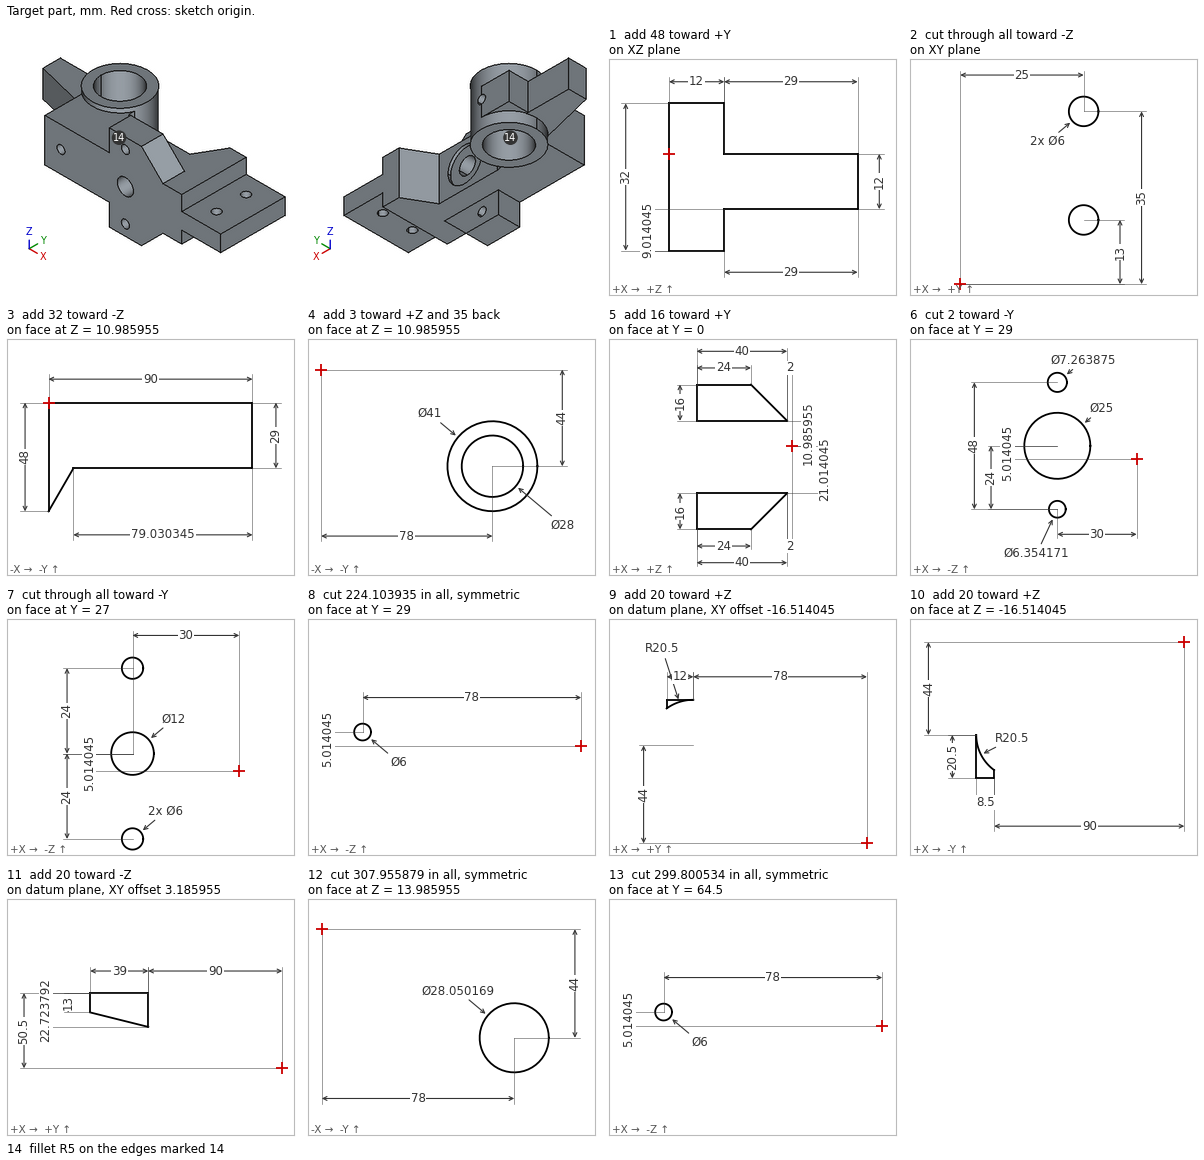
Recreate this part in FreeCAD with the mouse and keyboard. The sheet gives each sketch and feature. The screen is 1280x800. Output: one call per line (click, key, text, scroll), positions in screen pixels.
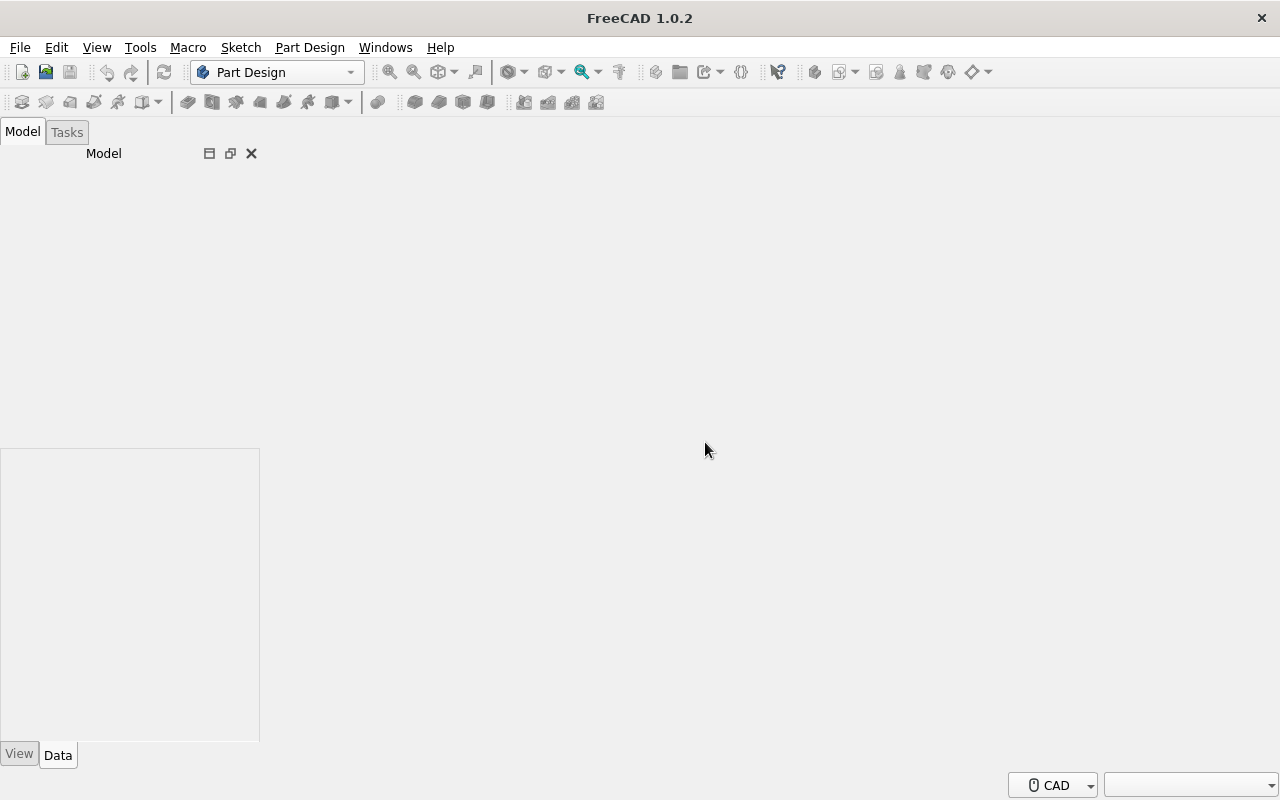
click(22, 72)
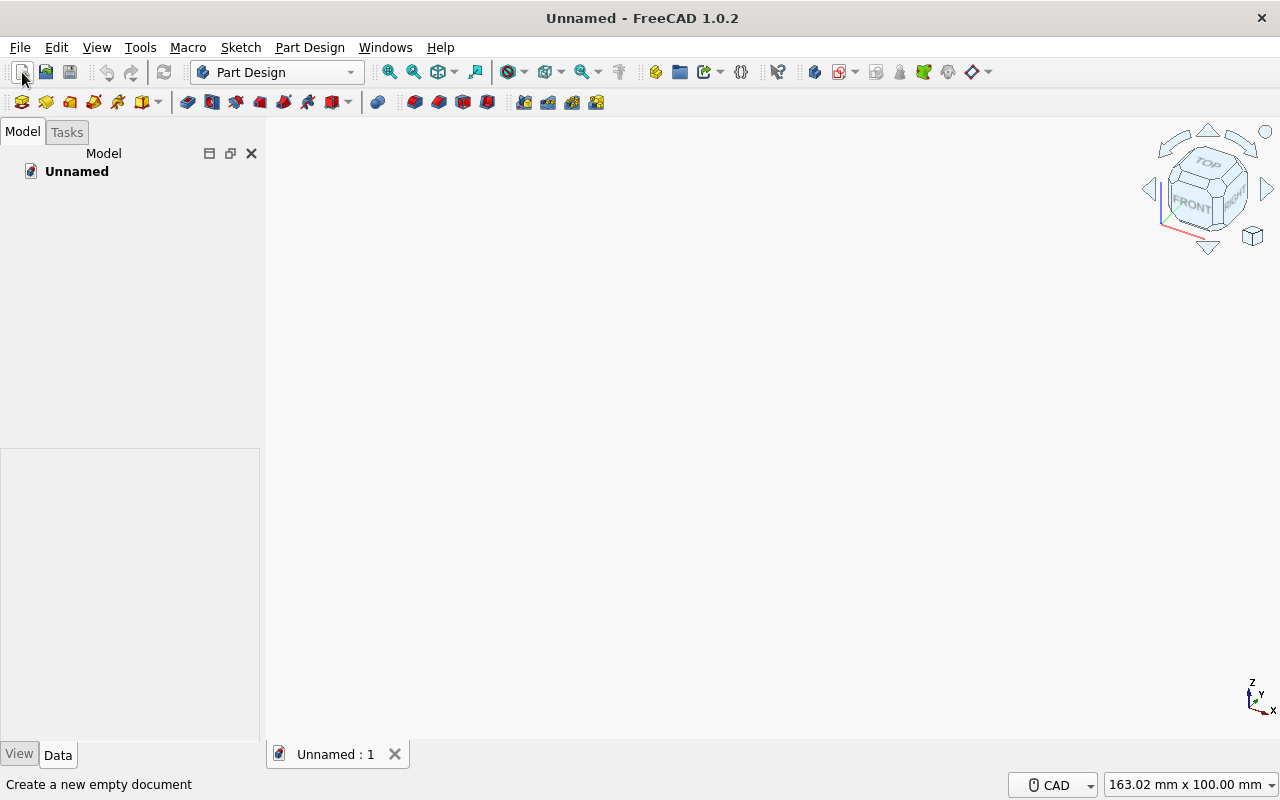
click(840, 72)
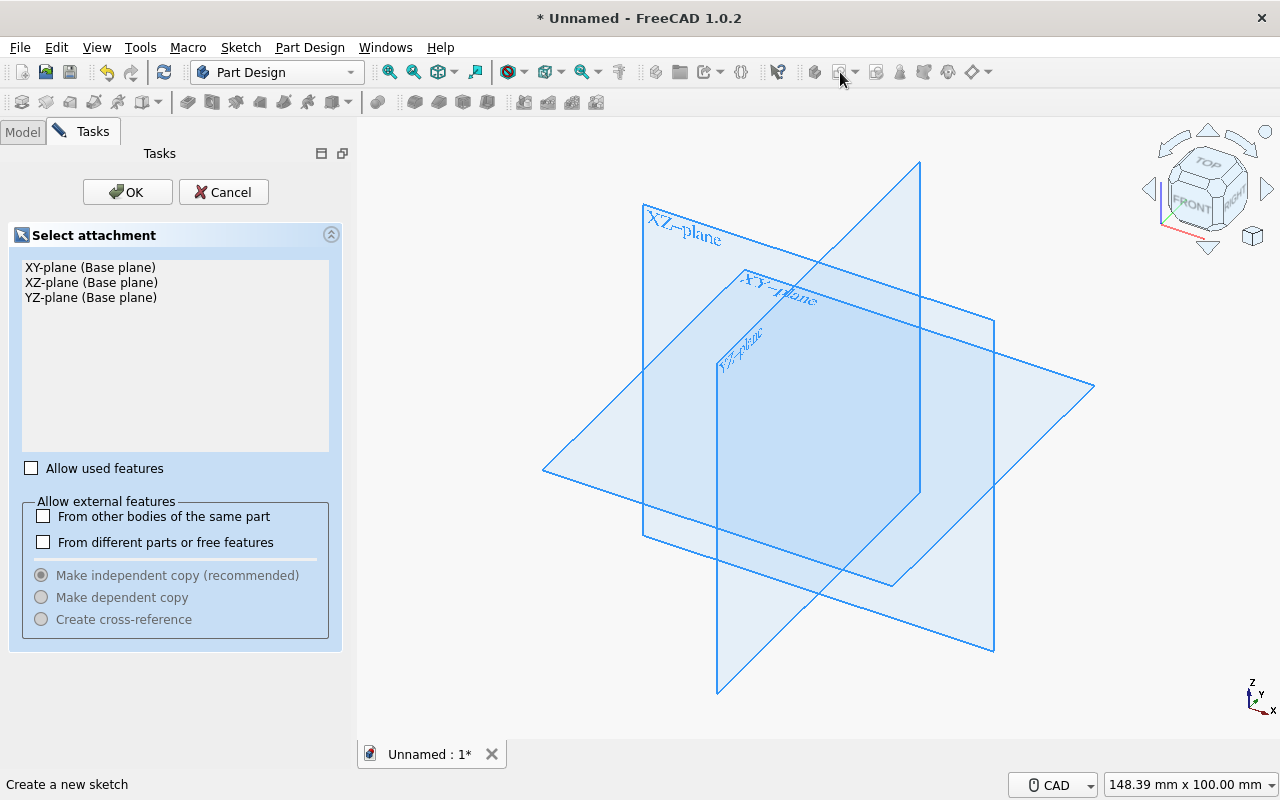
click(82, 282)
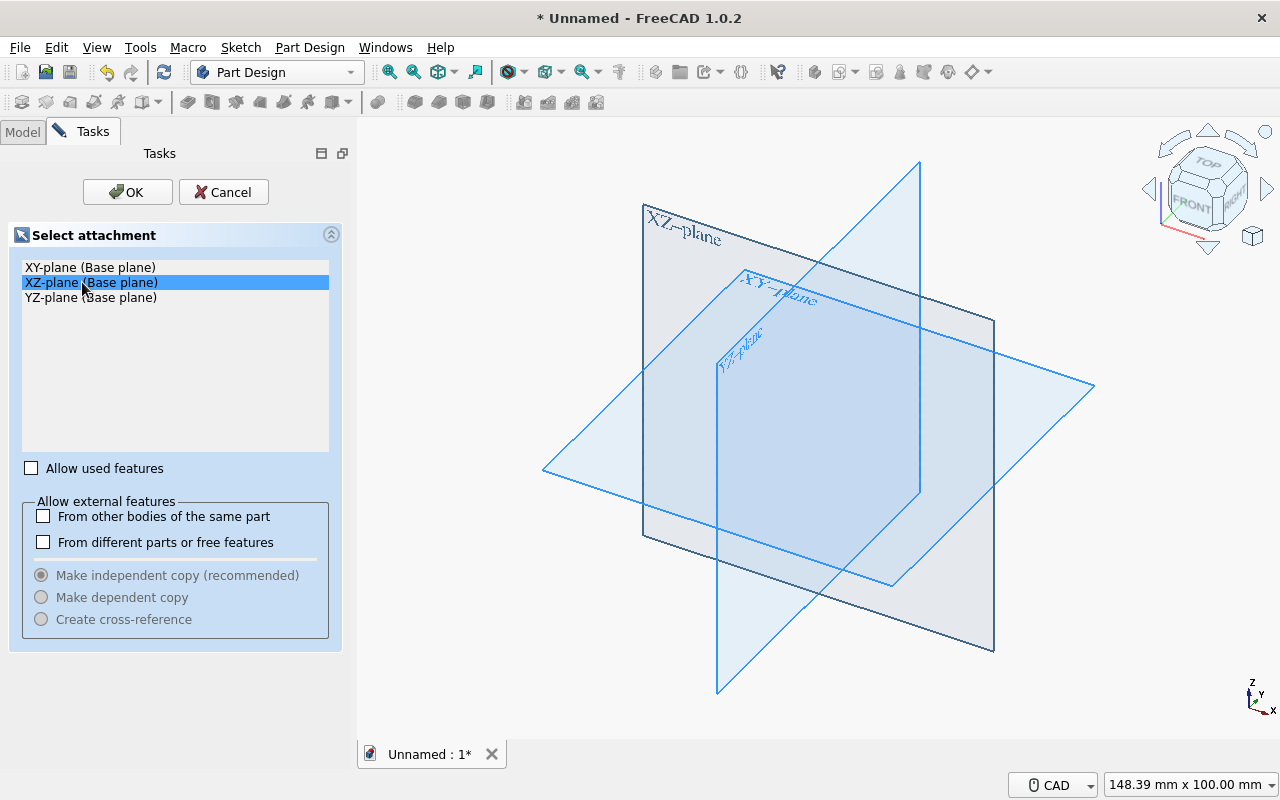
click(128, 192)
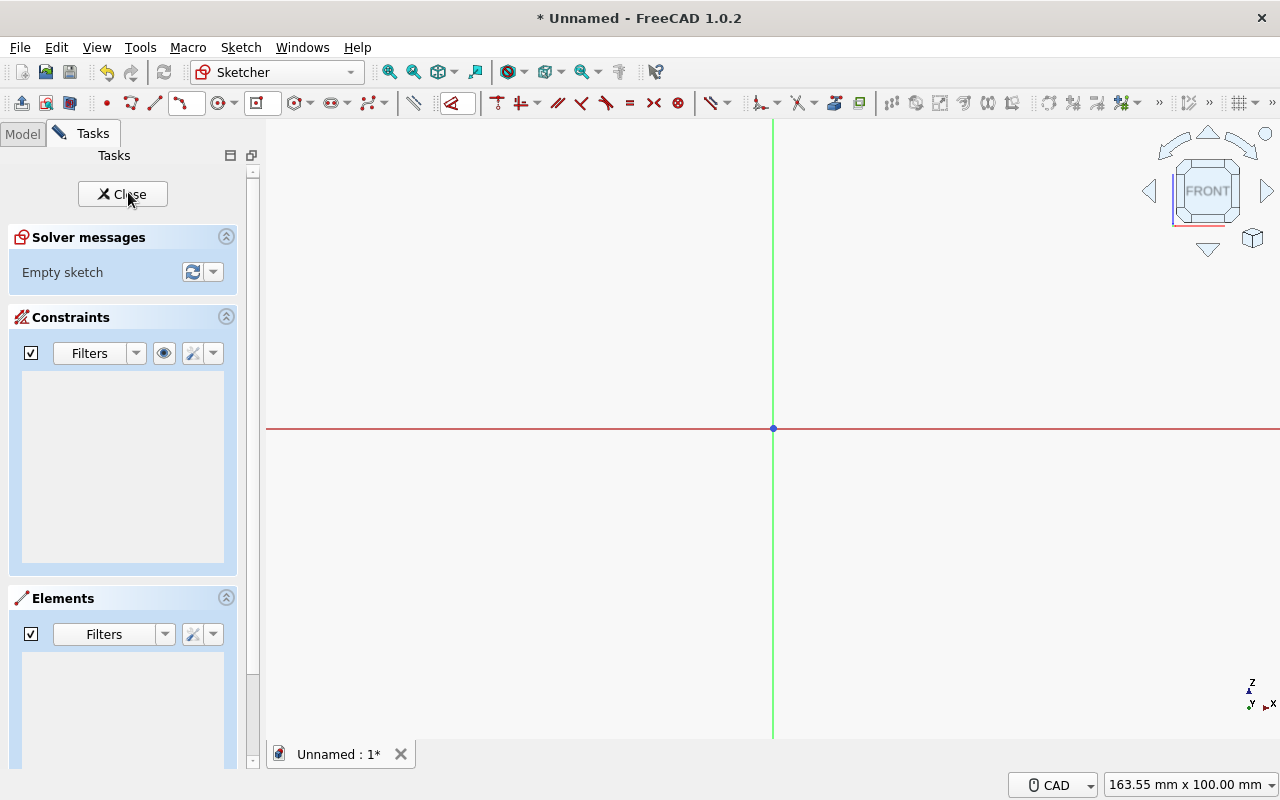
scroll(1115, 498, up, 3)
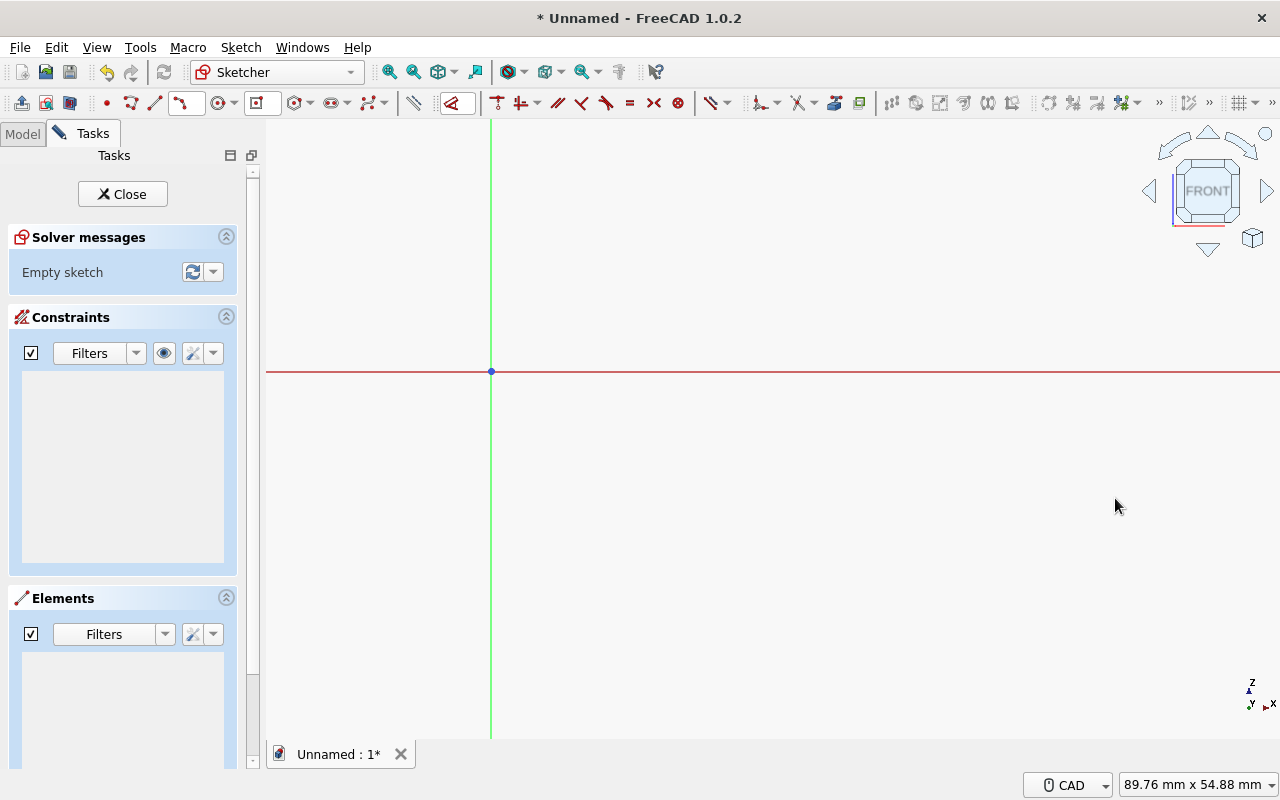
key(g)
key(m)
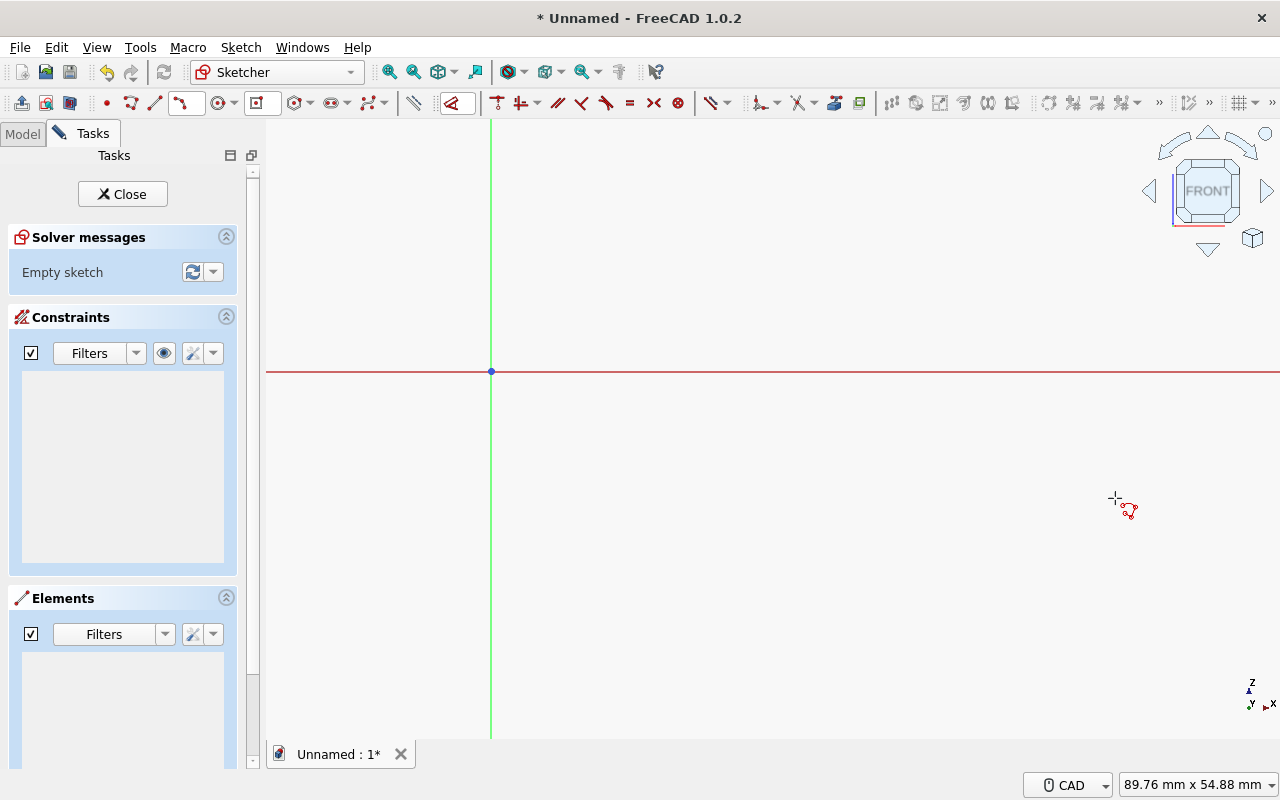
click(491, 248)
click(627, 248)
click(627, 372)
click(954, 381)
click(954, 507)
click(627, 507)
click(627, 609)
click(500, 609)
click(491, 249)
key(Escape)
key(Escape)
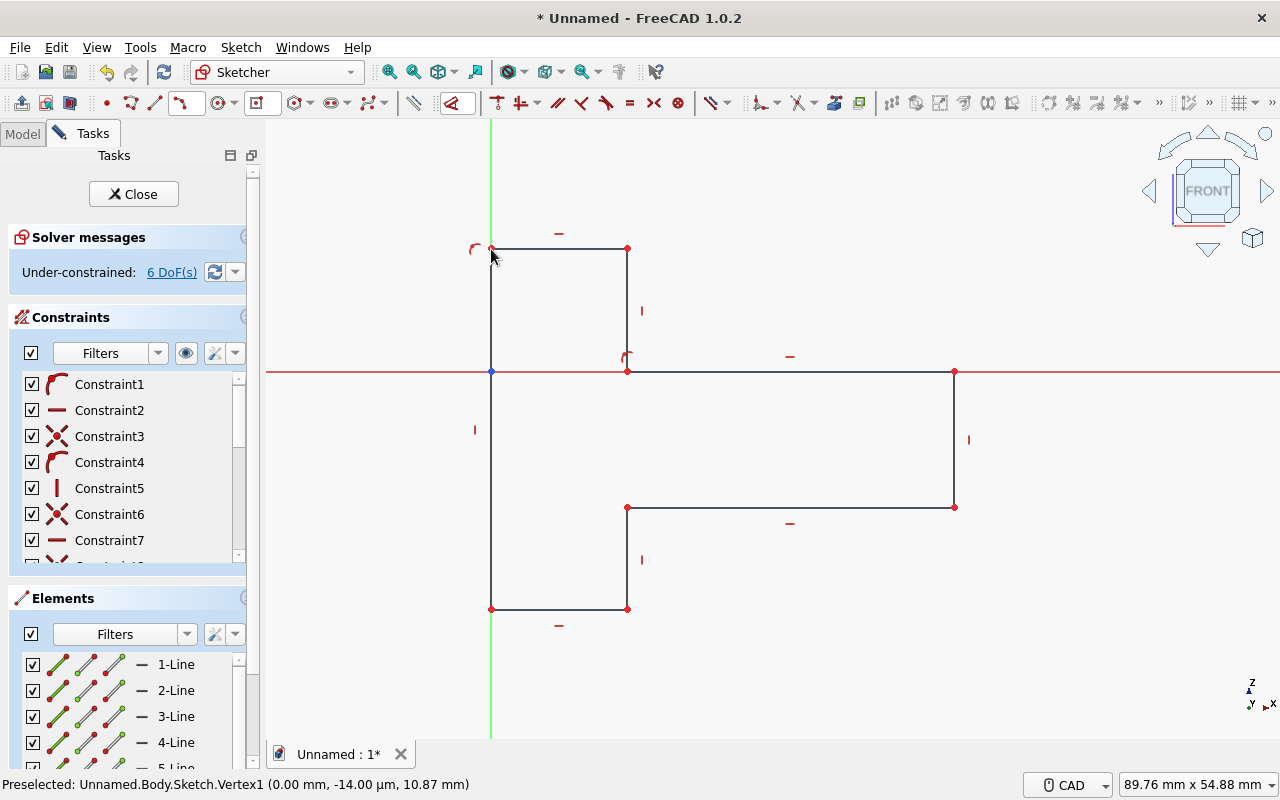
click(532, 249)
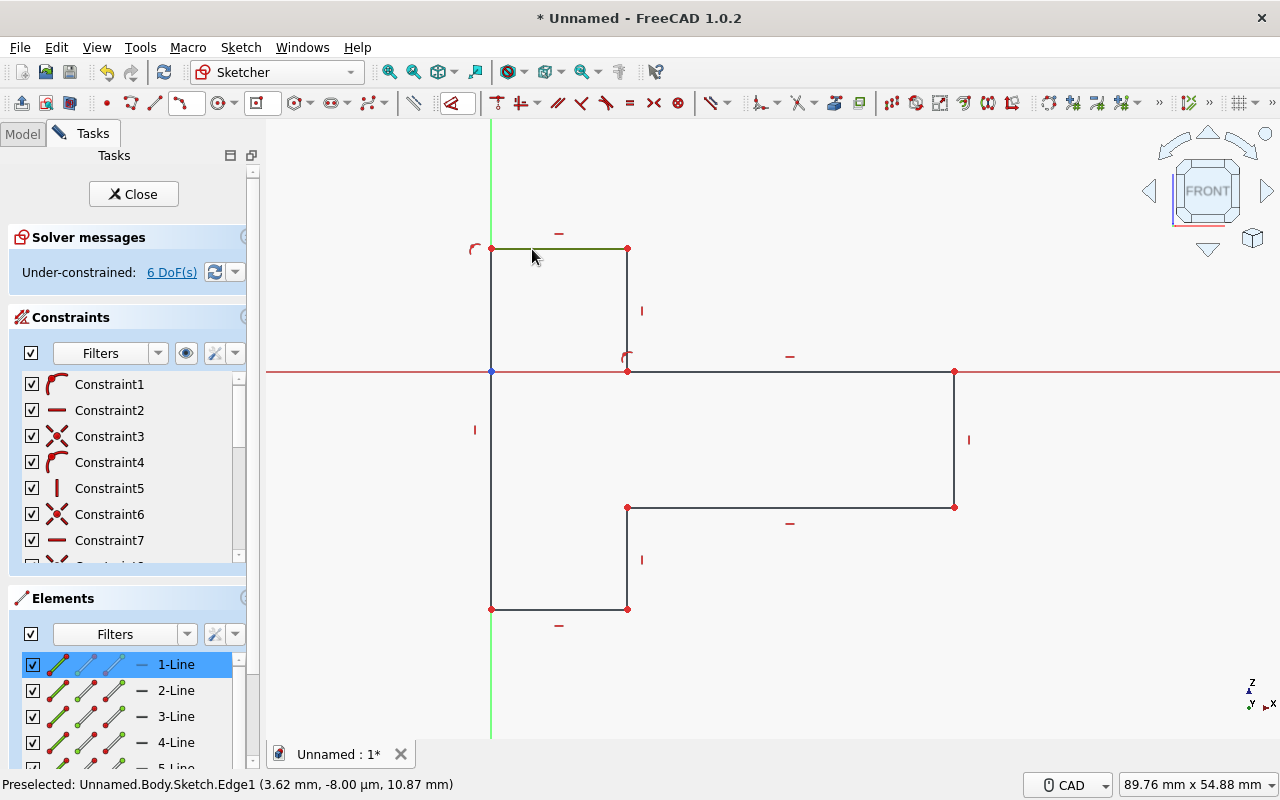
click(470, 104)